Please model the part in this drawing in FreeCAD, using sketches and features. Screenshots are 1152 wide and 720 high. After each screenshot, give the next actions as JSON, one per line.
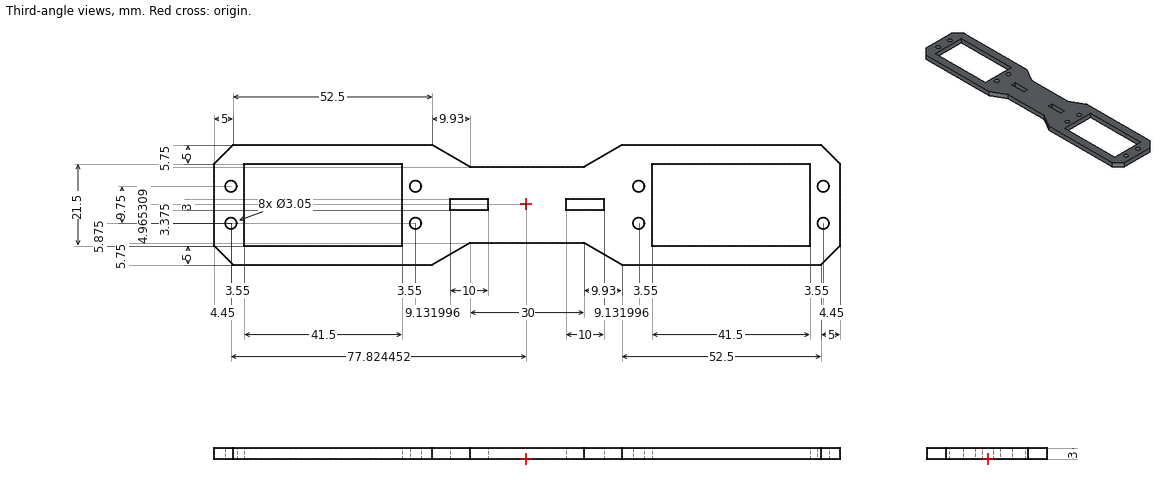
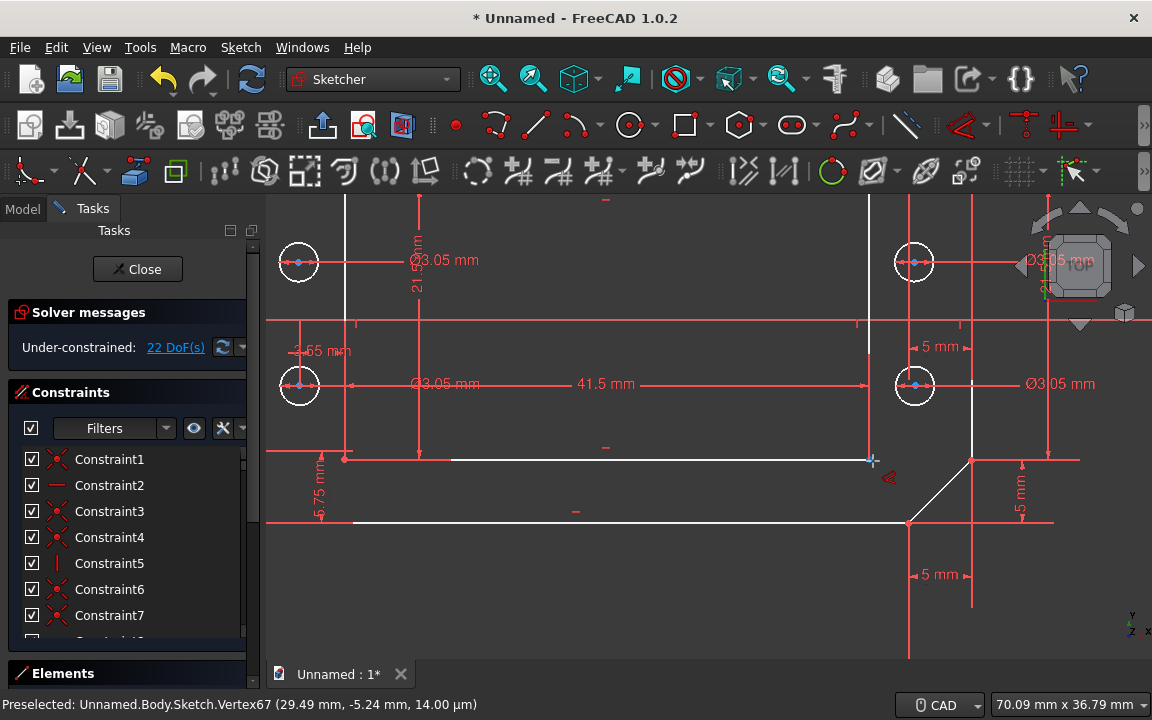
{"action": "left_click", "coordinate": [869, 460]}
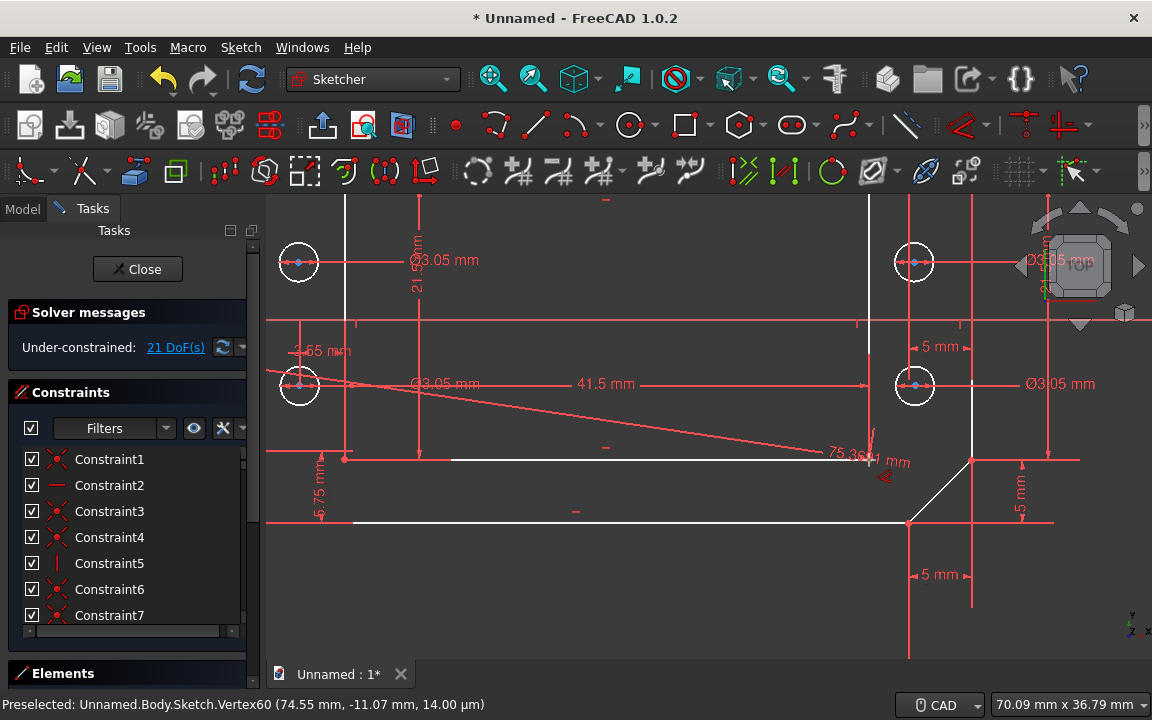
{"action": "left_click", "coordinate": [915, 386]}
{"action": "left_click", "coordinate": [892, 494]}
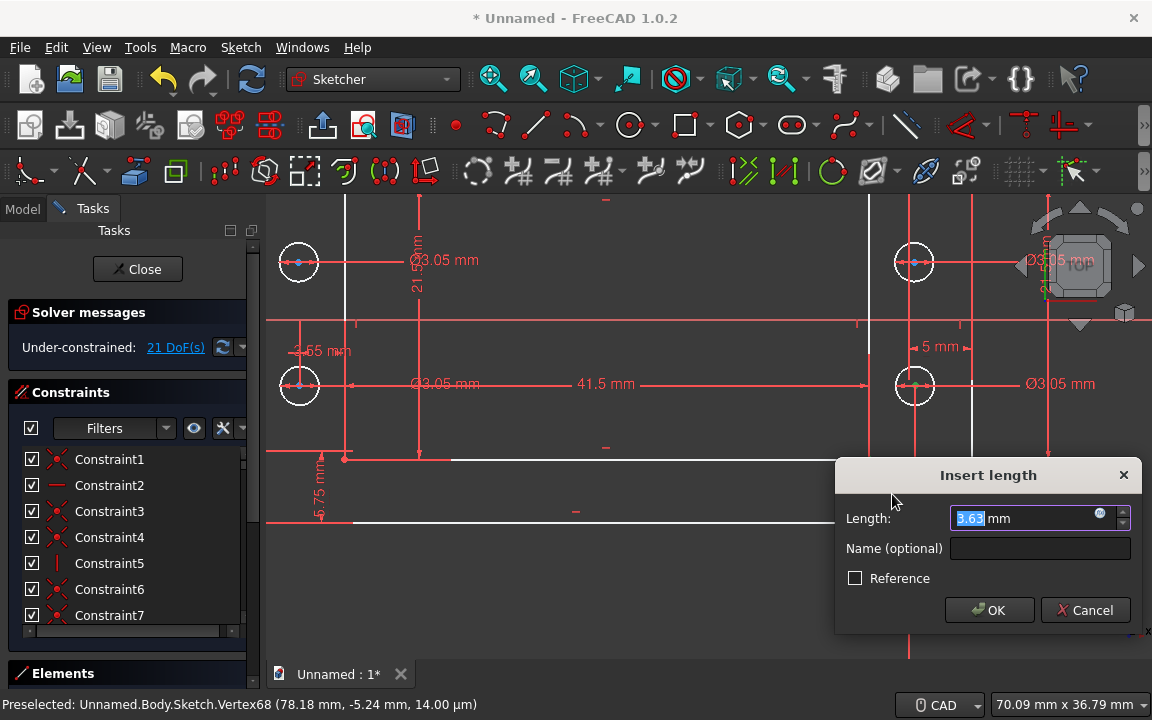
{"action": "type", "text": "3.55"}
{"action": "key", "text": "Return"}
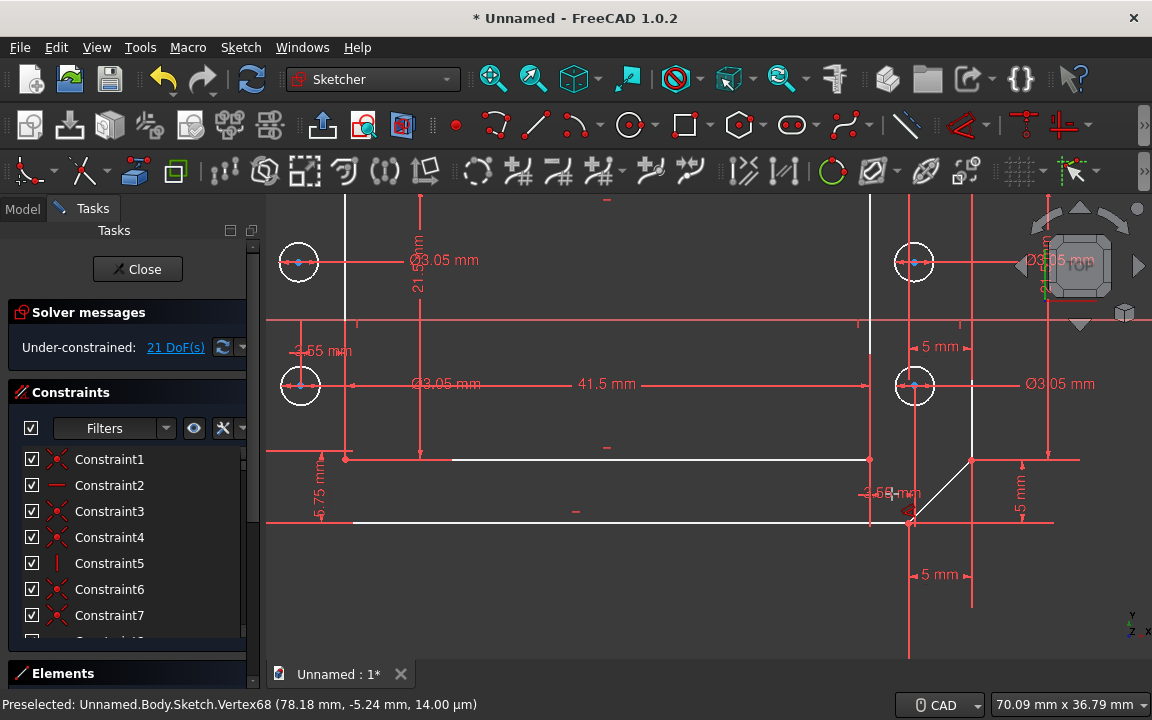
{"action": "left_click", "coordinate": [972, 460]}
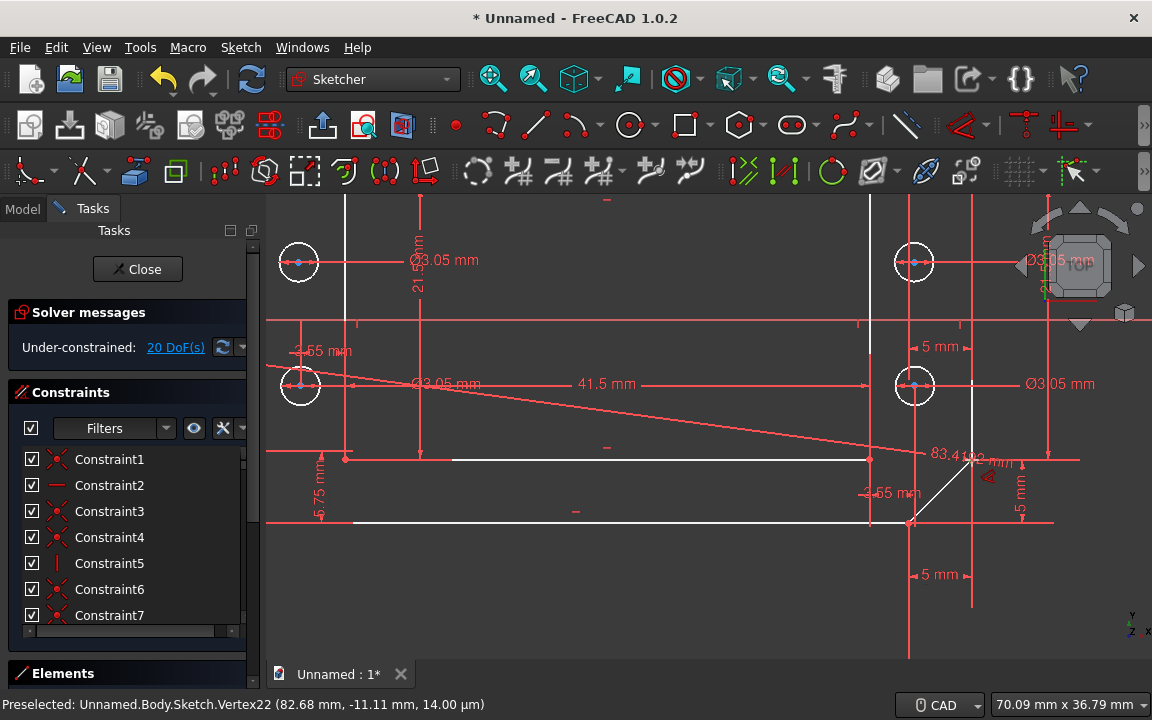
{"action": "left_click", "coordinate": [915, 386]}
{"action": "left_click", "coordinate": [943, 518]}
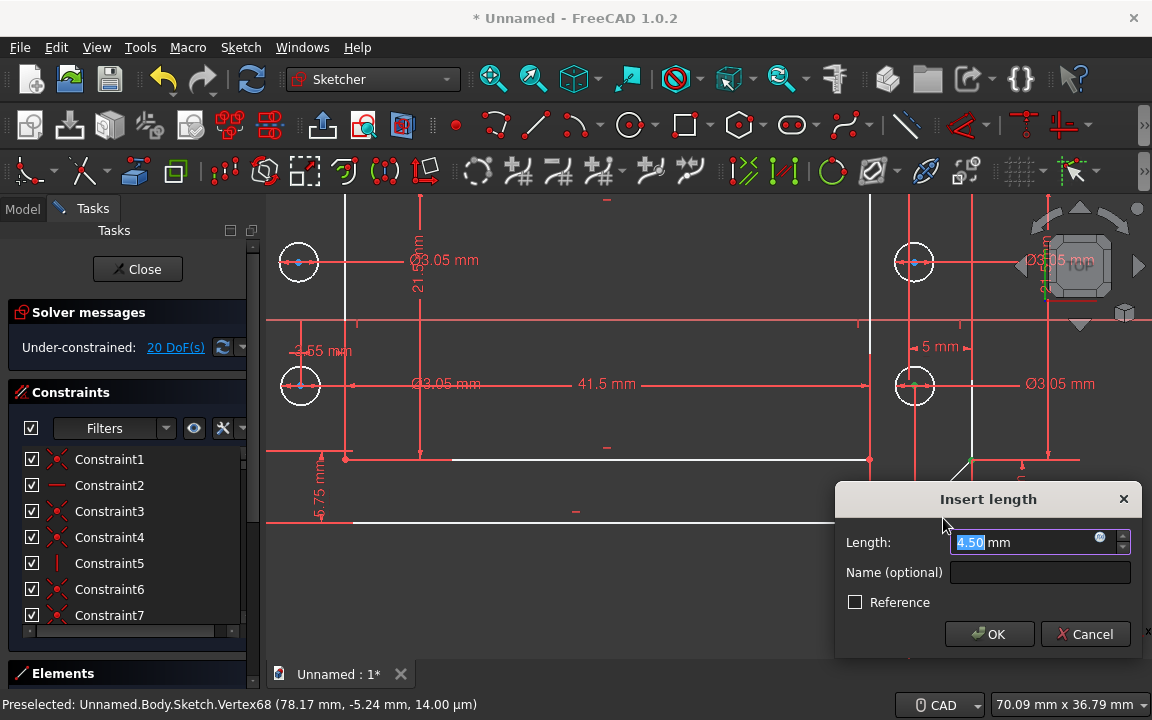
{"action": "type", "text": "4.45"}
{"action": "key", "text": "Return"}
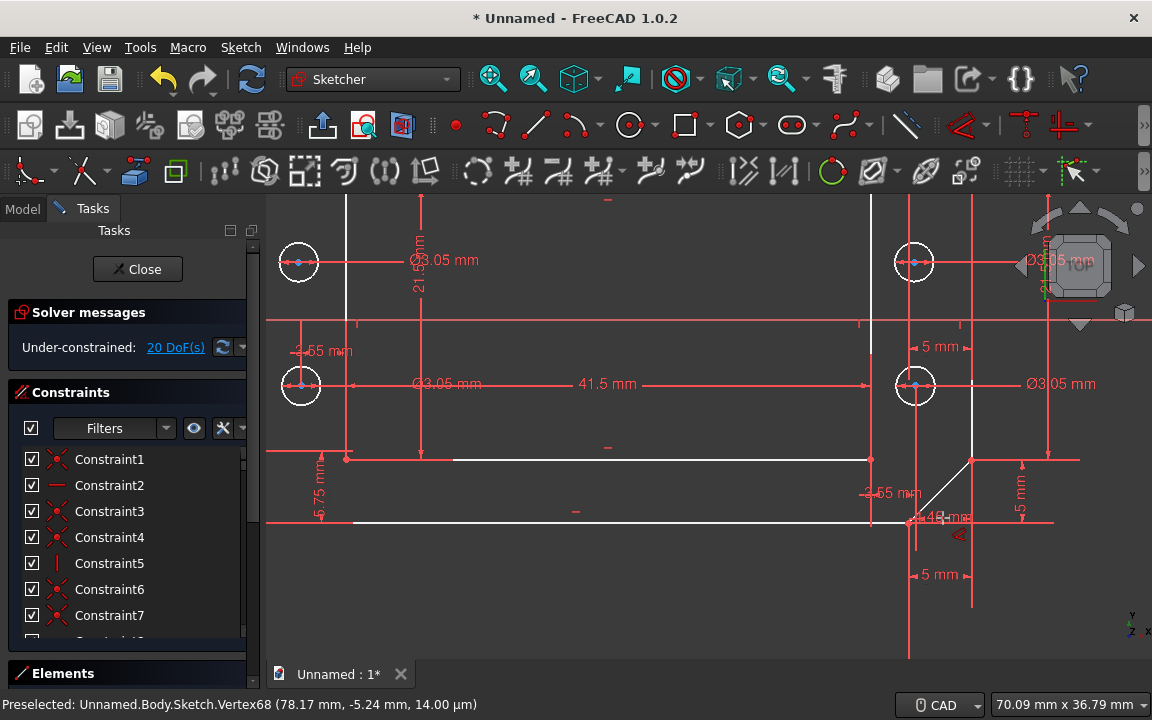
{"action": "scroll", "coordinate": [873, 461], "scroll_direction": "down", "scroll_amount": 7}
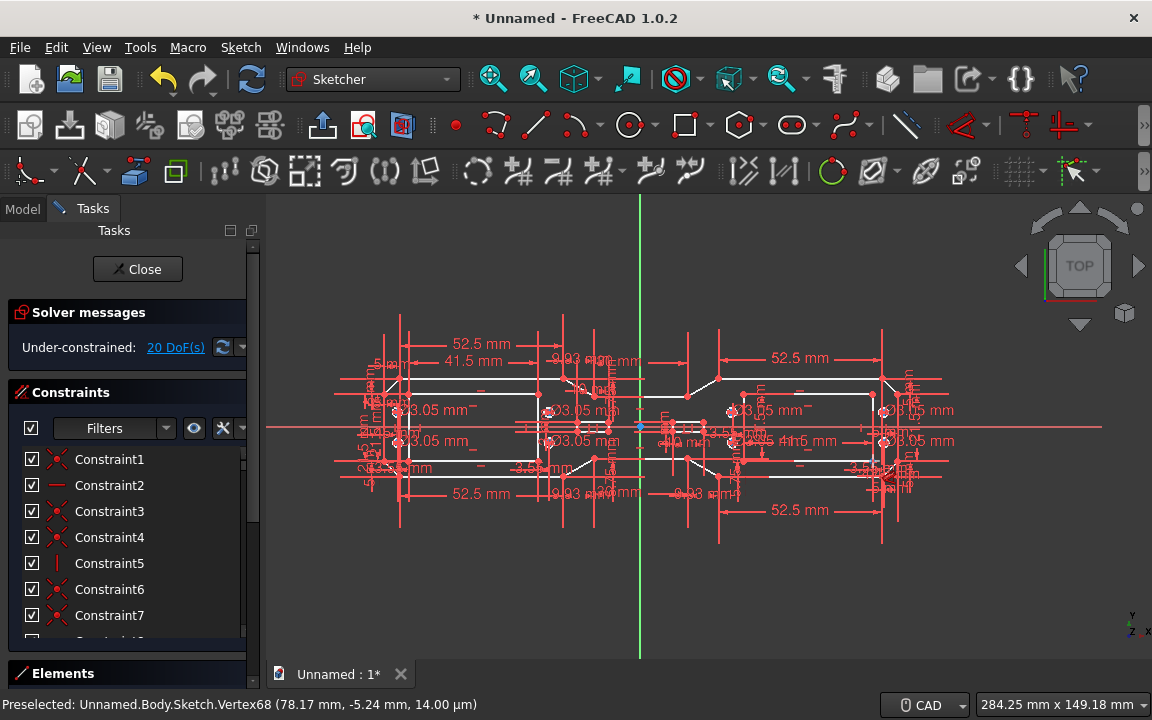
{"action": "scroll", "coordinate": [409, 394], "scroll_direction": "up", "scroll_amount": 7}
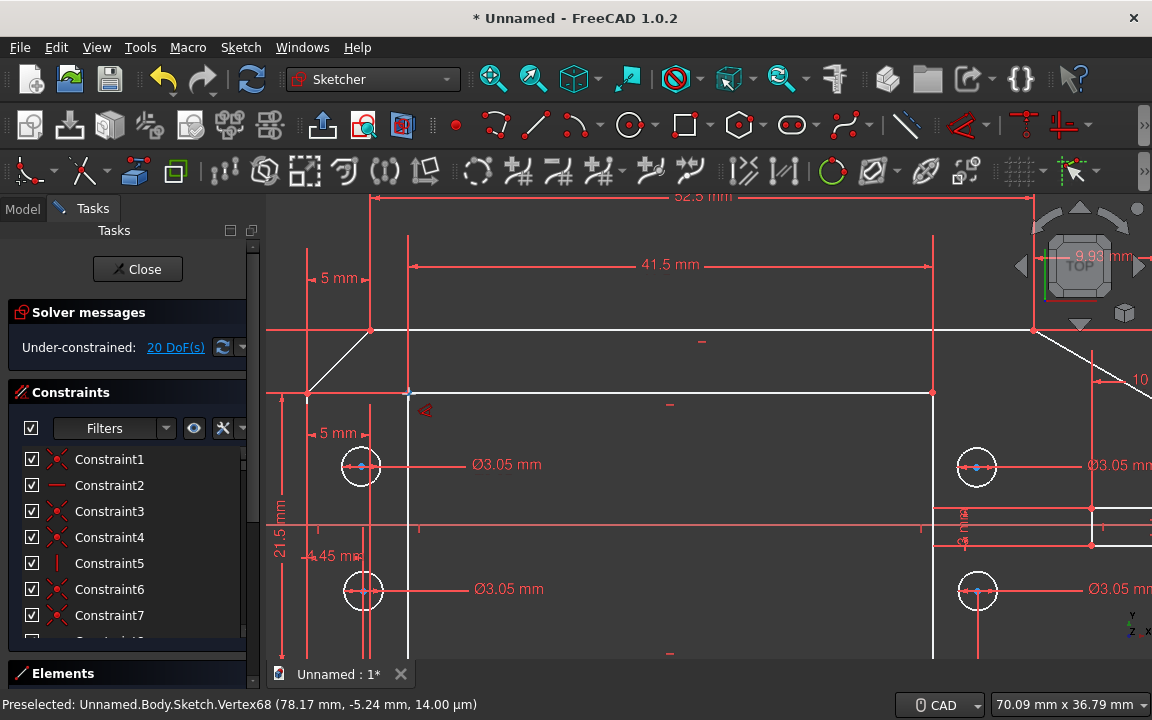
{"action": "left_click", "coordinate": [408, 393]}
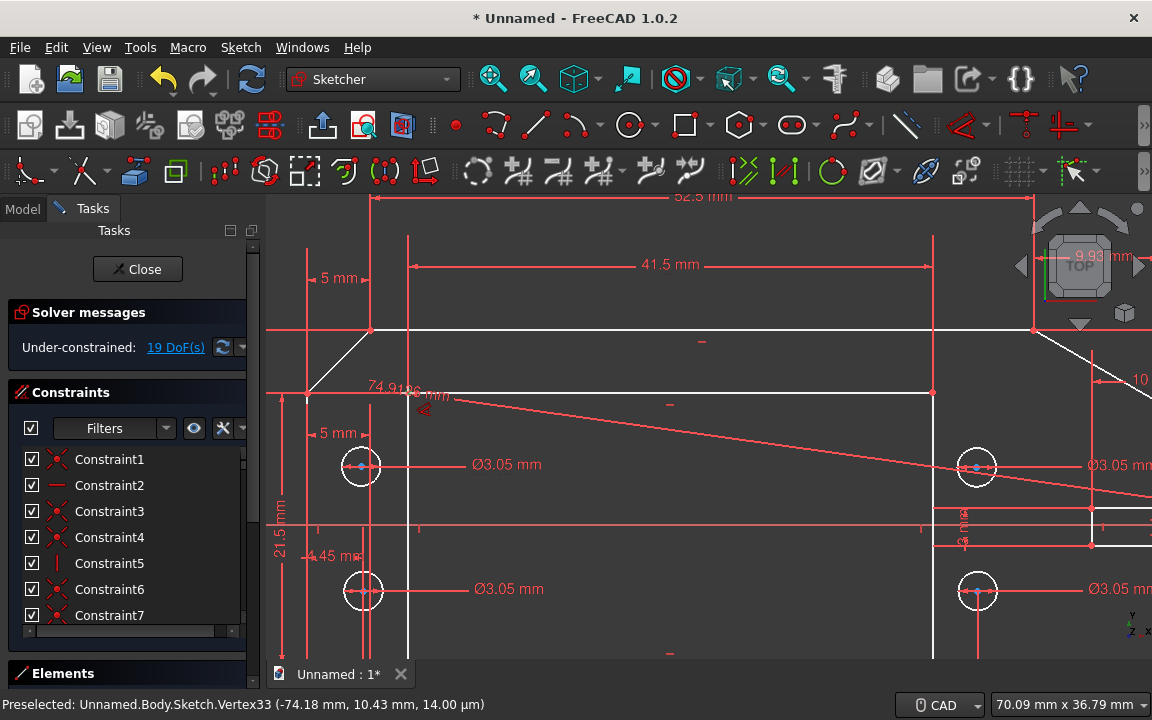
{"action": "left_click", "coordinate": [361, 467]}
{"action": "left_click", "coordinate": [385, 359]}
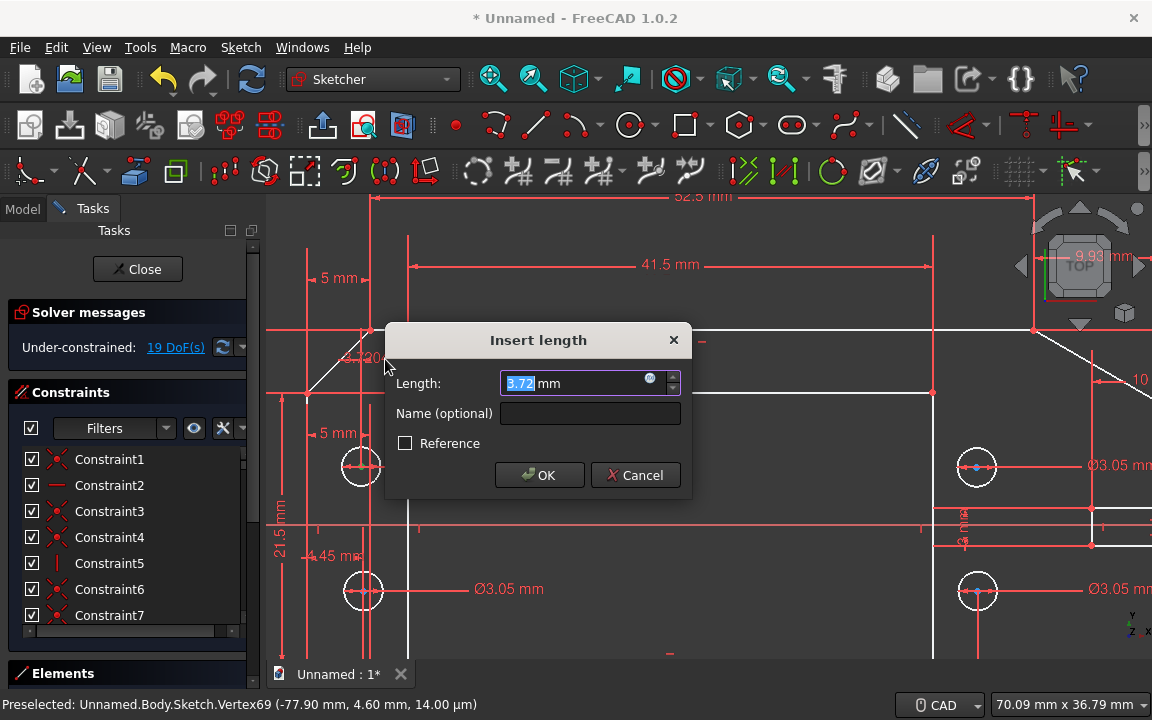
{"action": "type", "text": "3.55"}
{"action": "key", "text": "Return"}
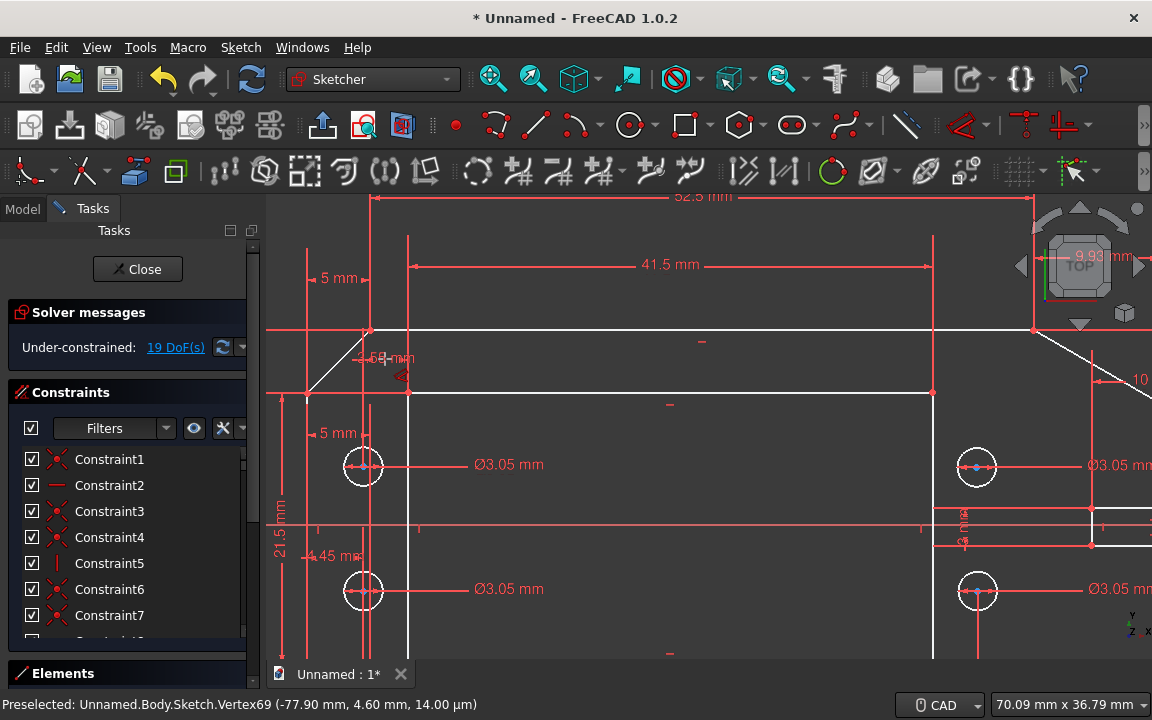
{"action": "scroll", "coordinate": [409, 394], "scroll_direction": "down", "scroll_amount": 7}